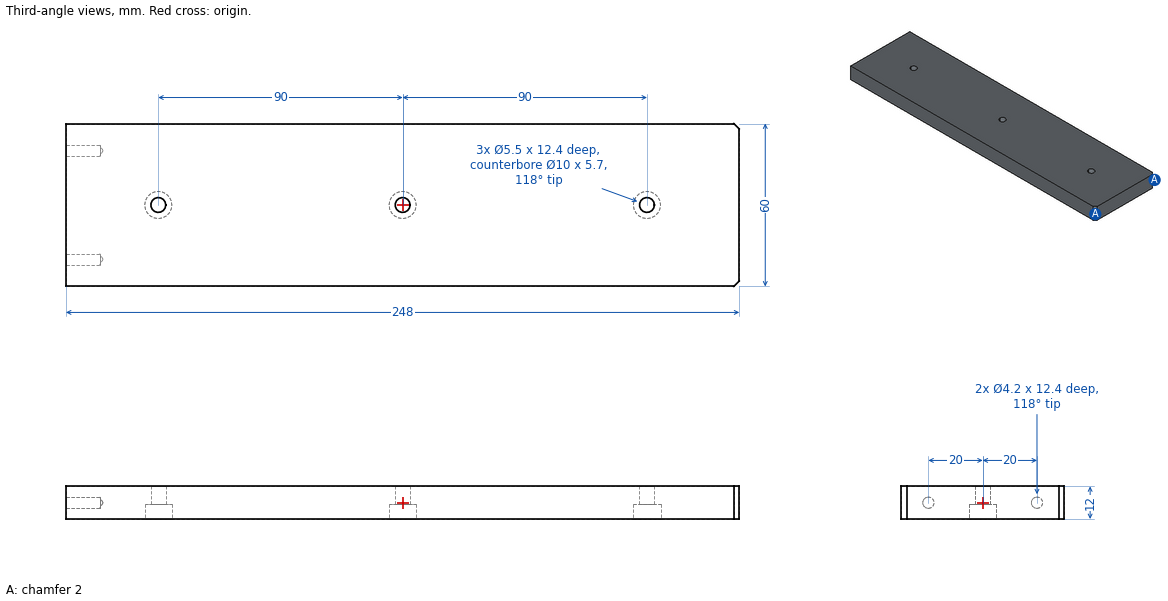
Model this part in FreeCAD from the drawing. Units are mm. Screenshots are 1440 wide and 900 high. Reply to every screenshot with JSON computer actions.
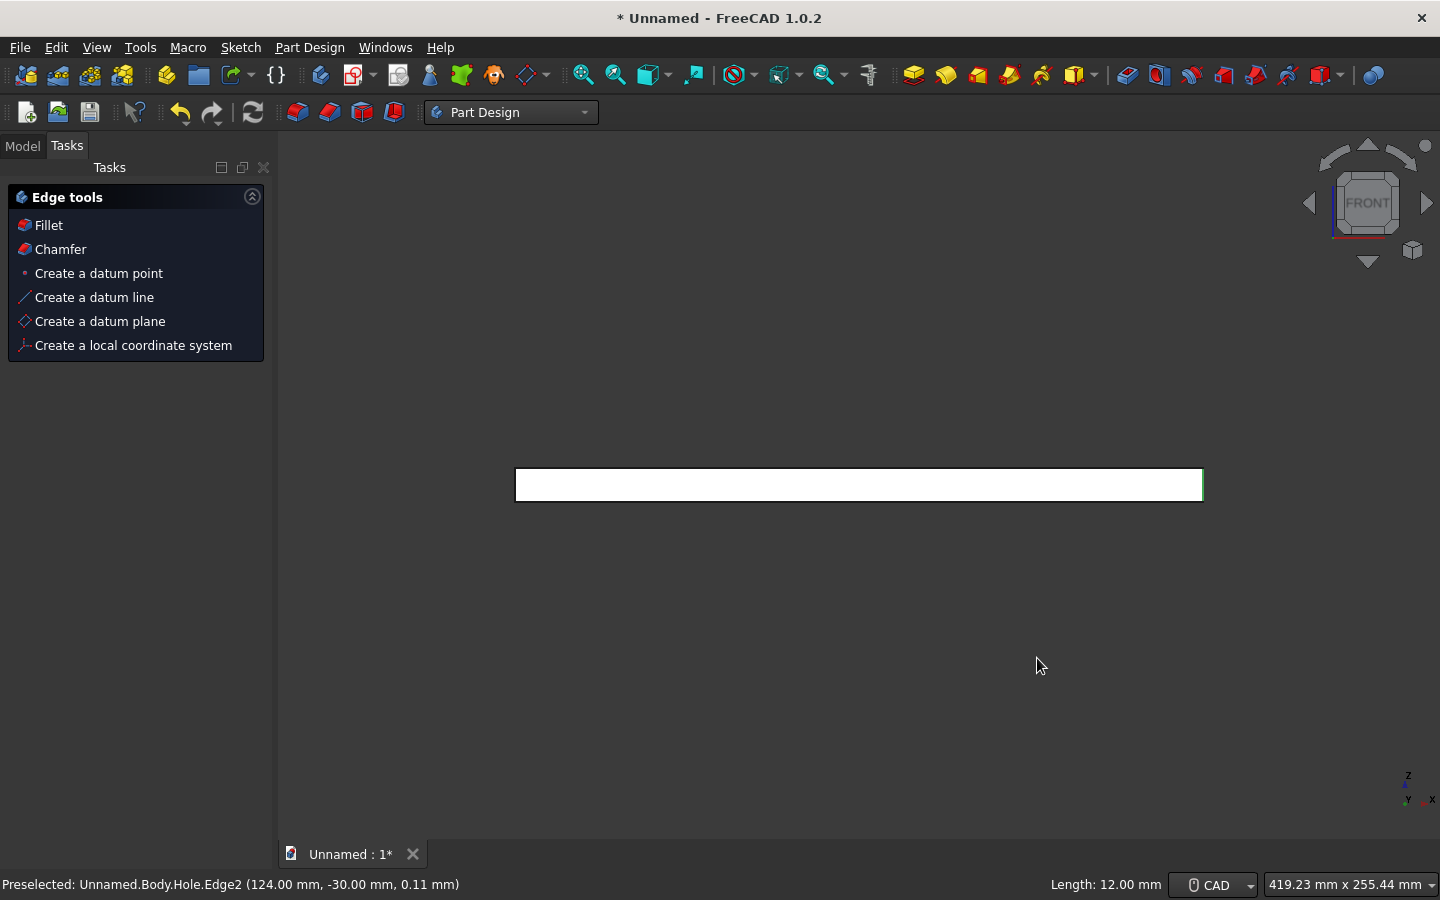
{"action": "key", "text": "3"}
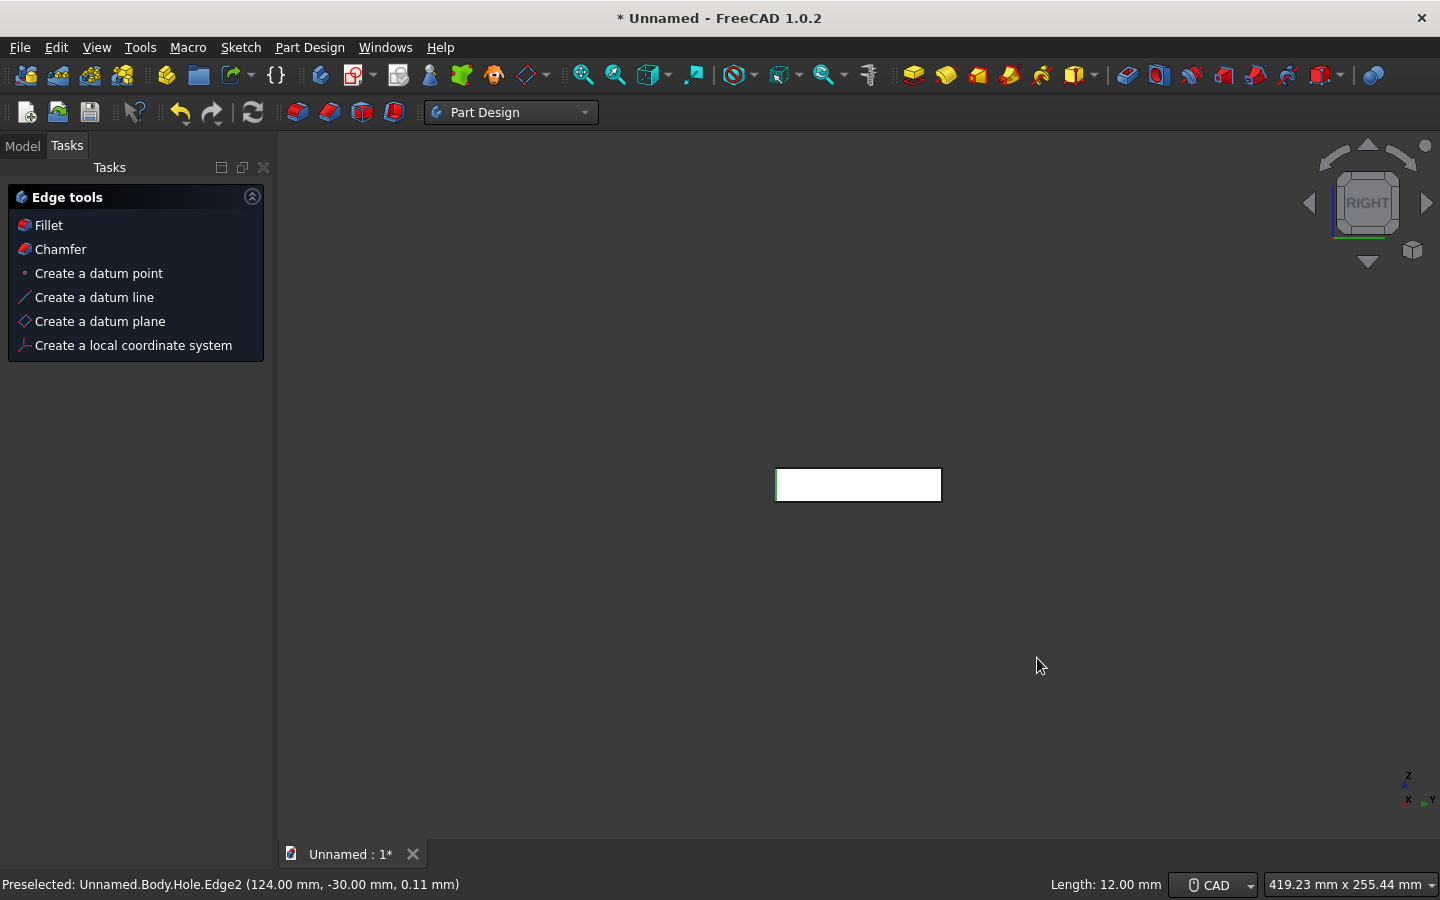
{"action": "left_click", "coordinate": [584, 76]}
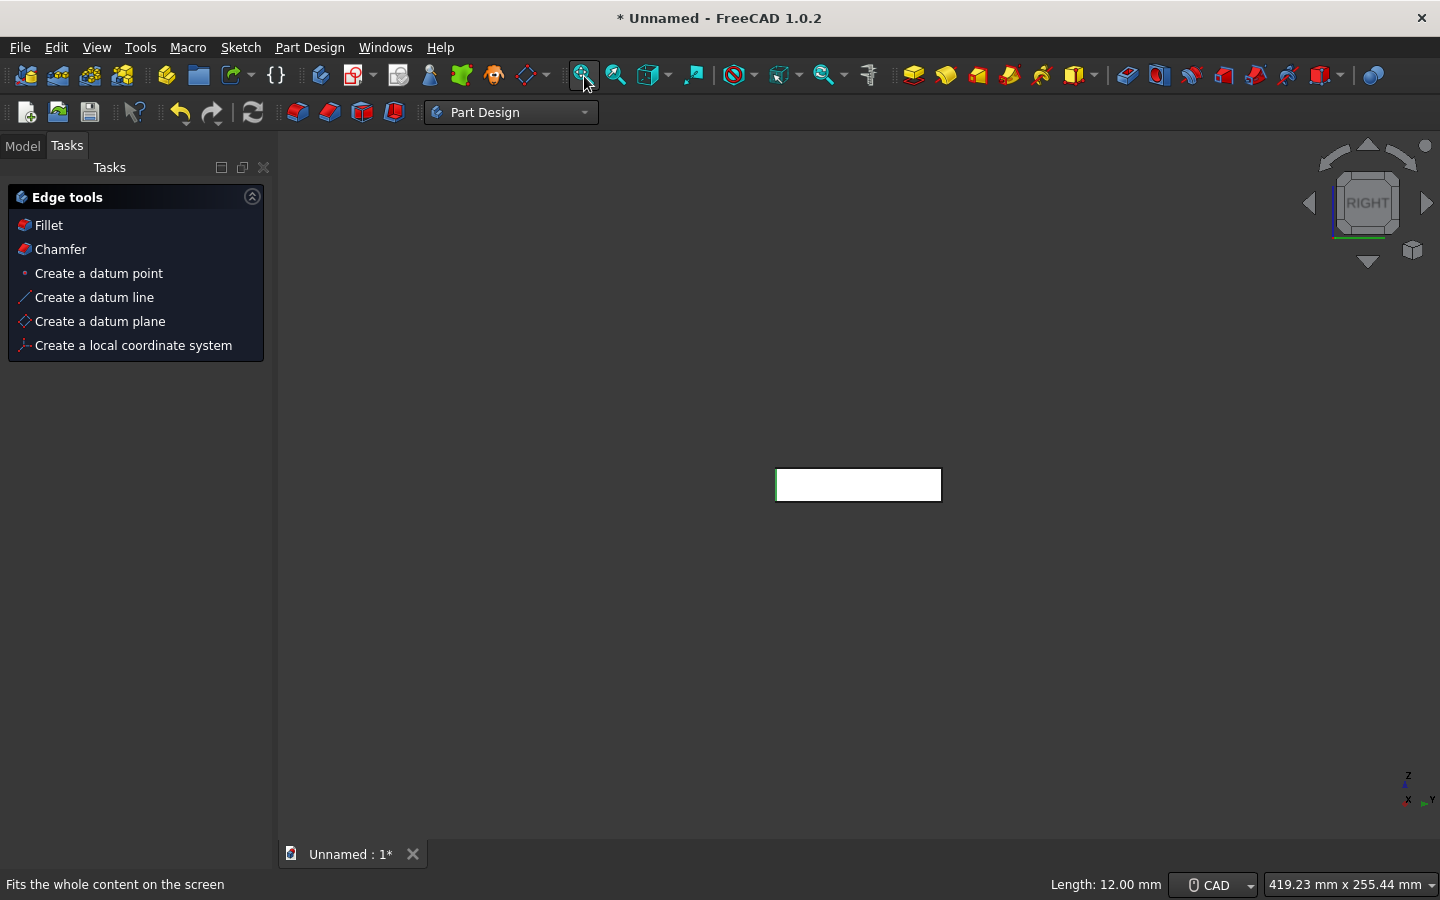
{"action": "left_click", "coordinate": [942, 484], "text": "ctrl"}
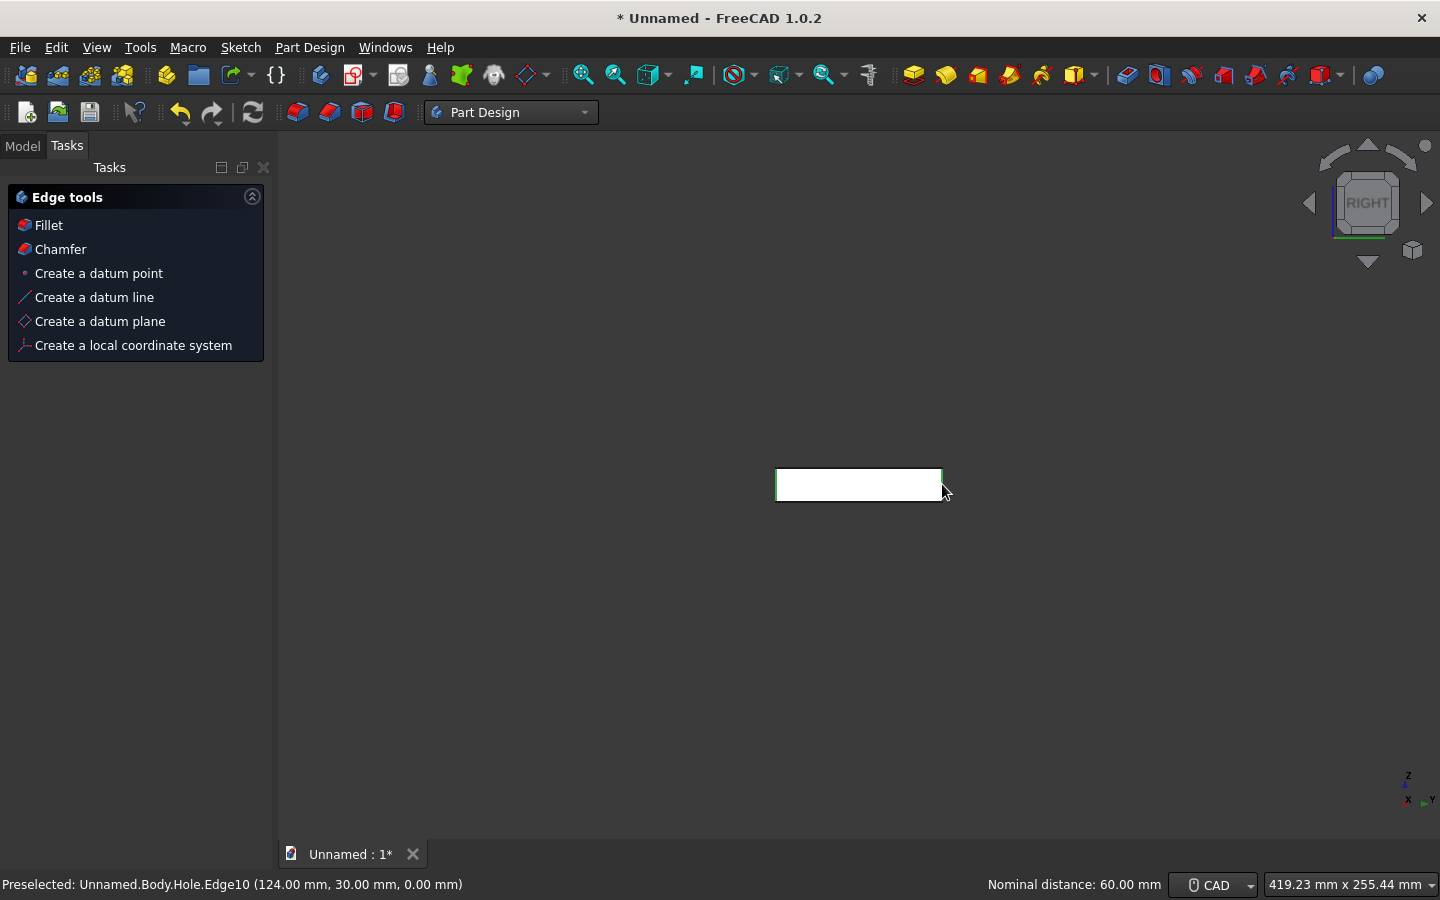
{"action": "left_click", "coordinate": [330, 112]}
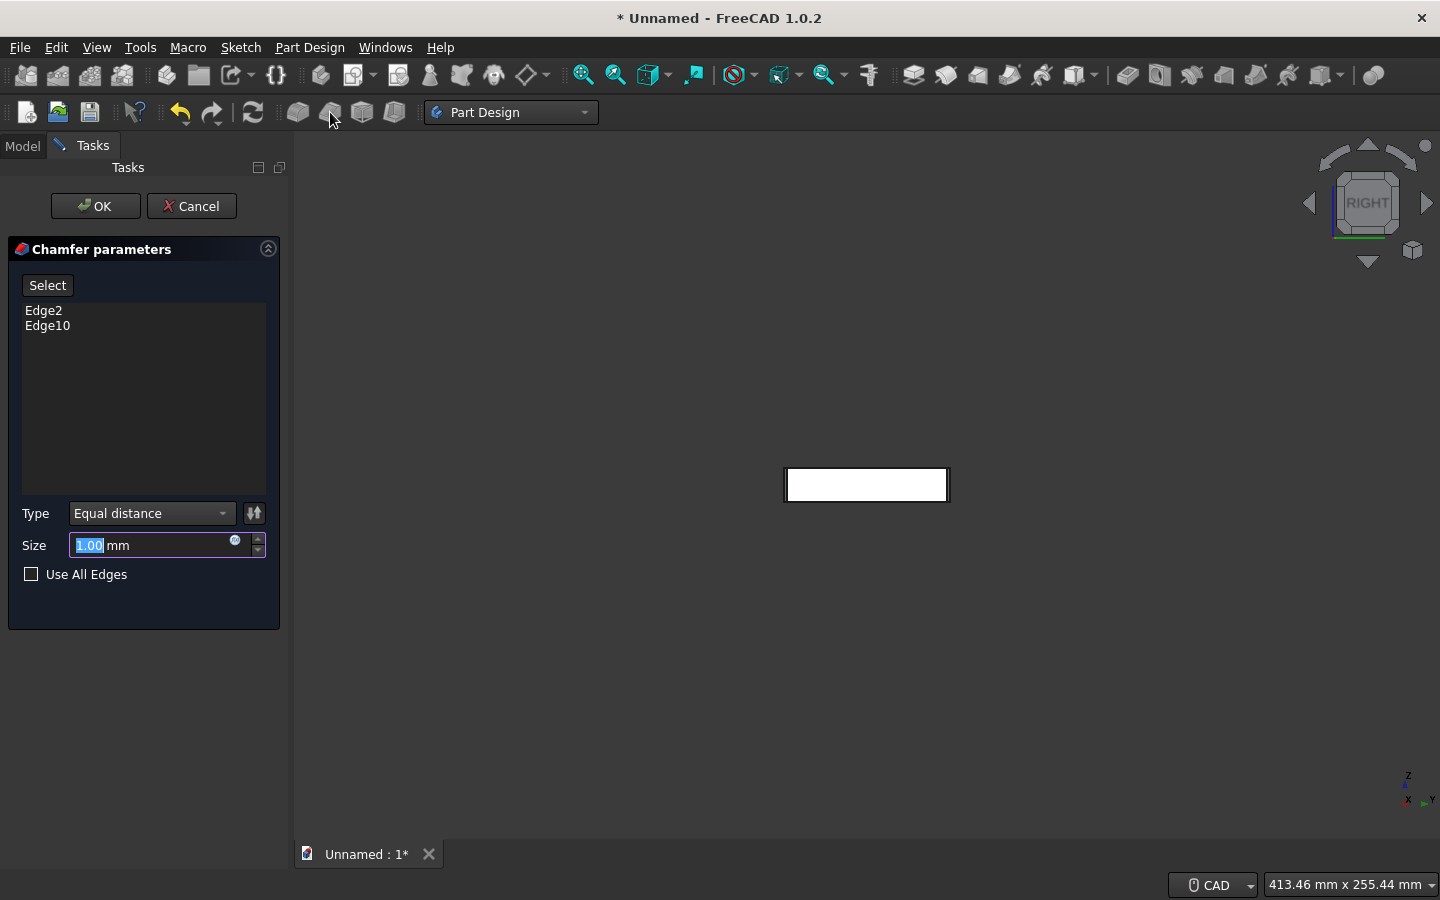
{"action": "type", "text": "2"}
{"action": "key", "text": "Tab"}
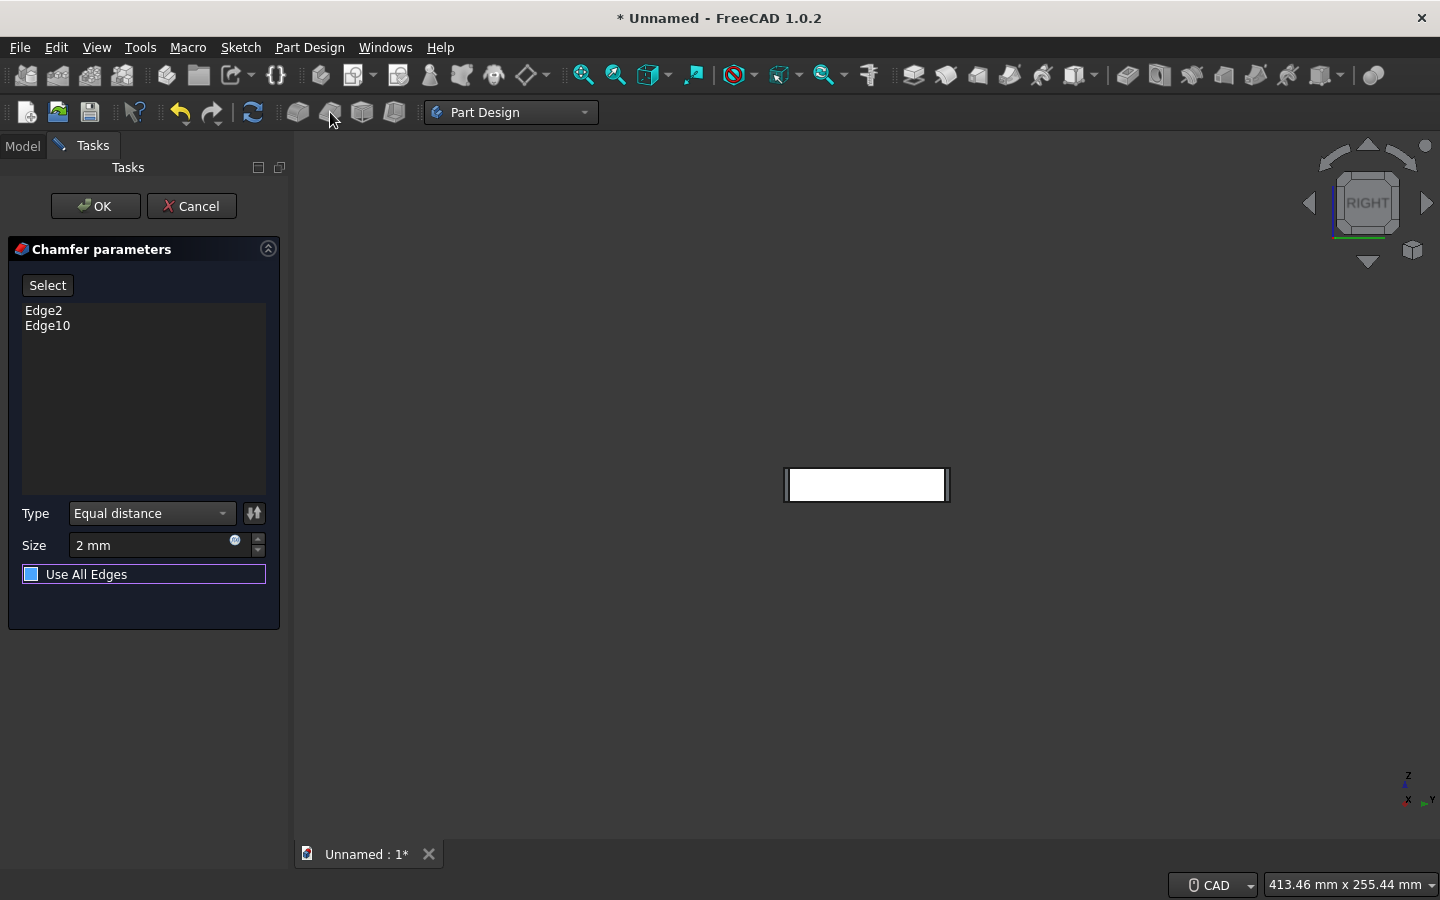
{"action": "left_click", "coordinate": [96, 206]}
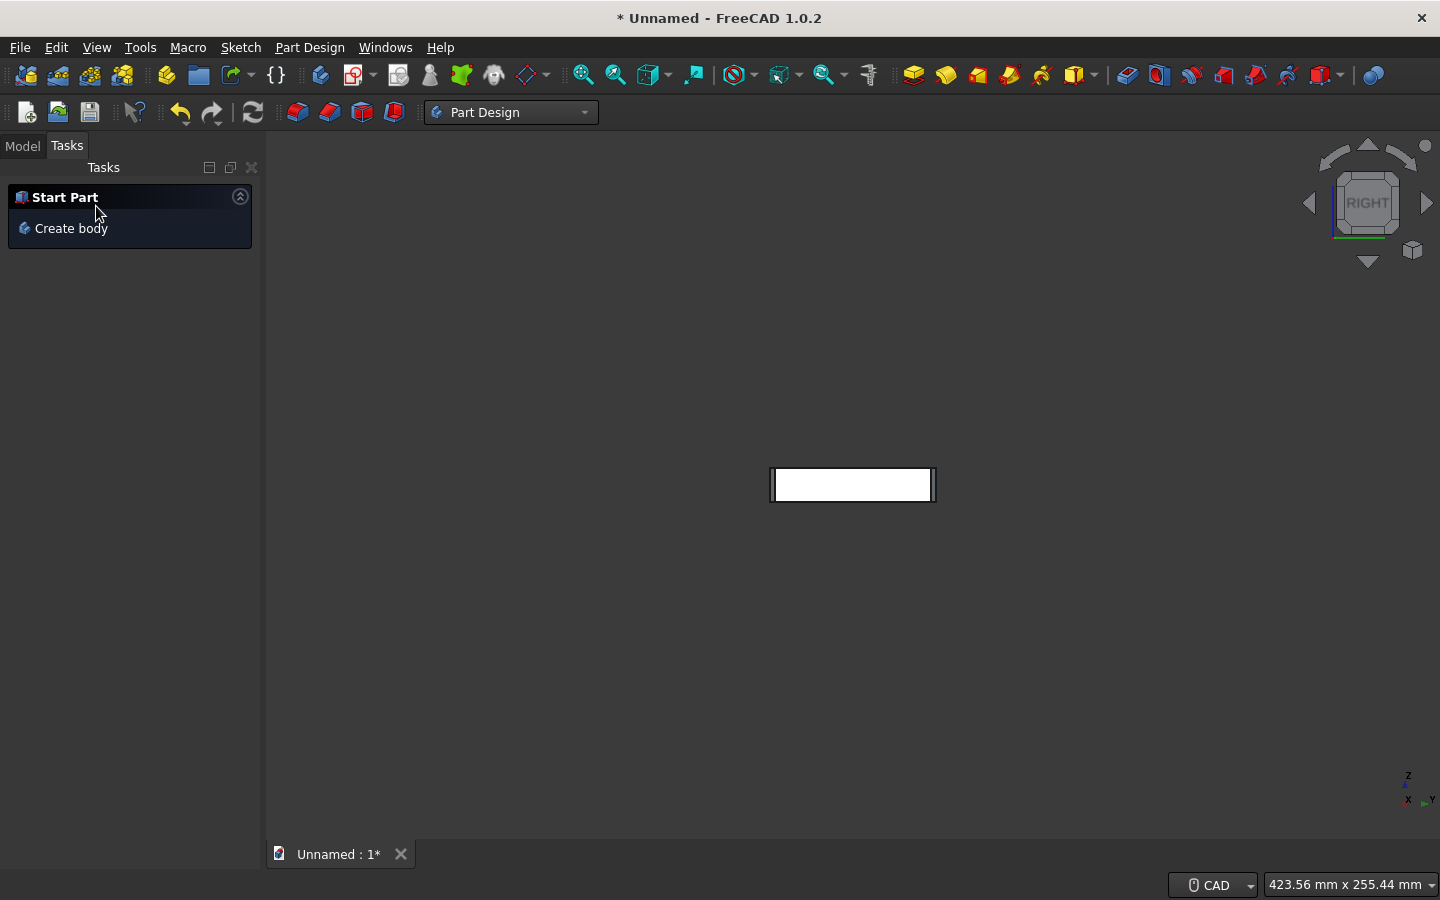
{"action": "left_click", "coordinate": [584, 76]}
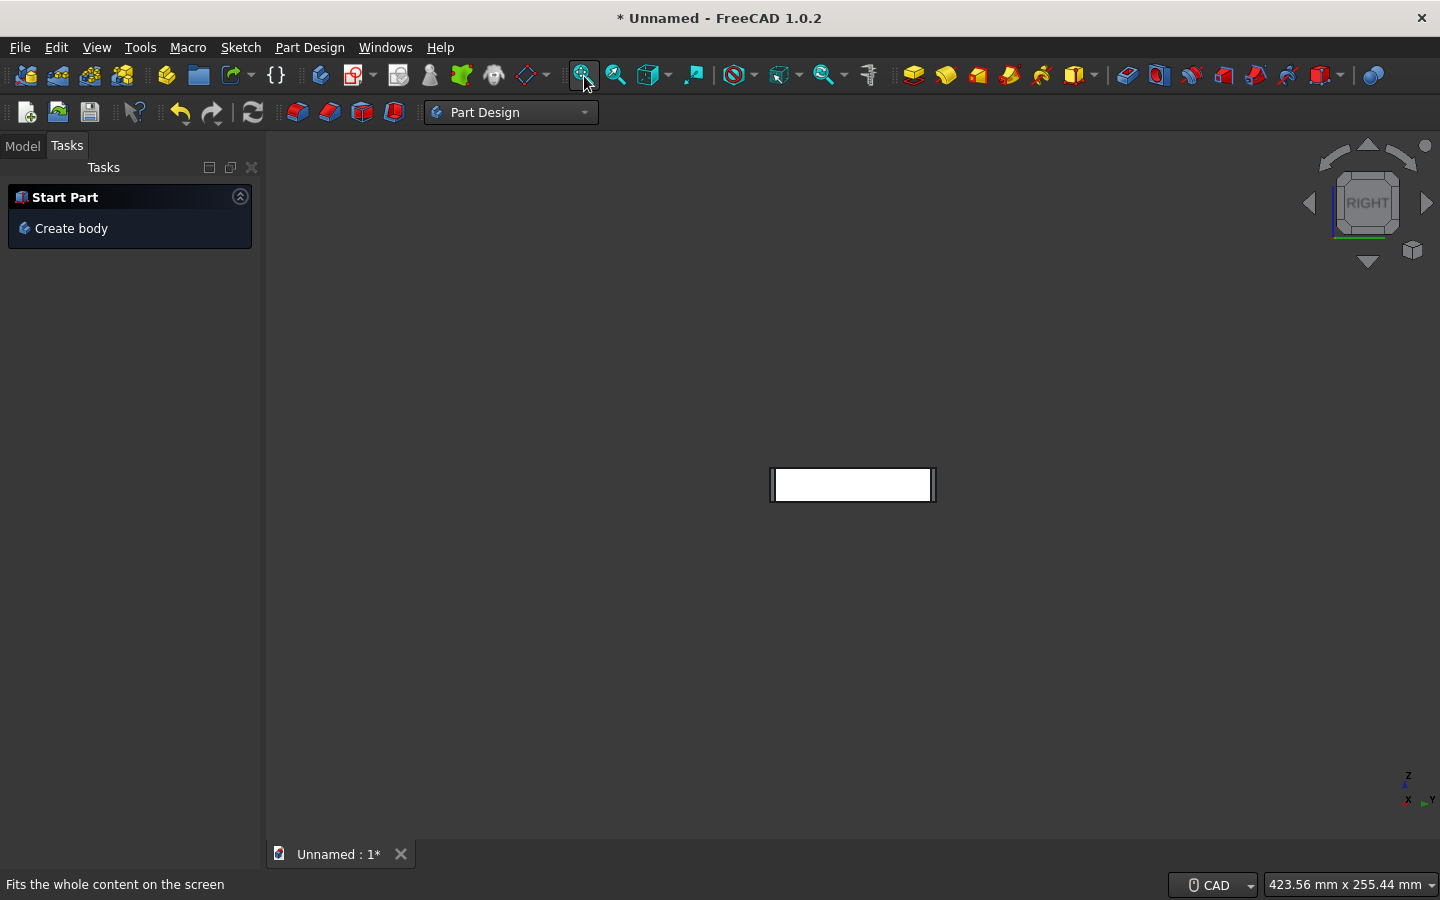
{"action": "key", "text": "5"}